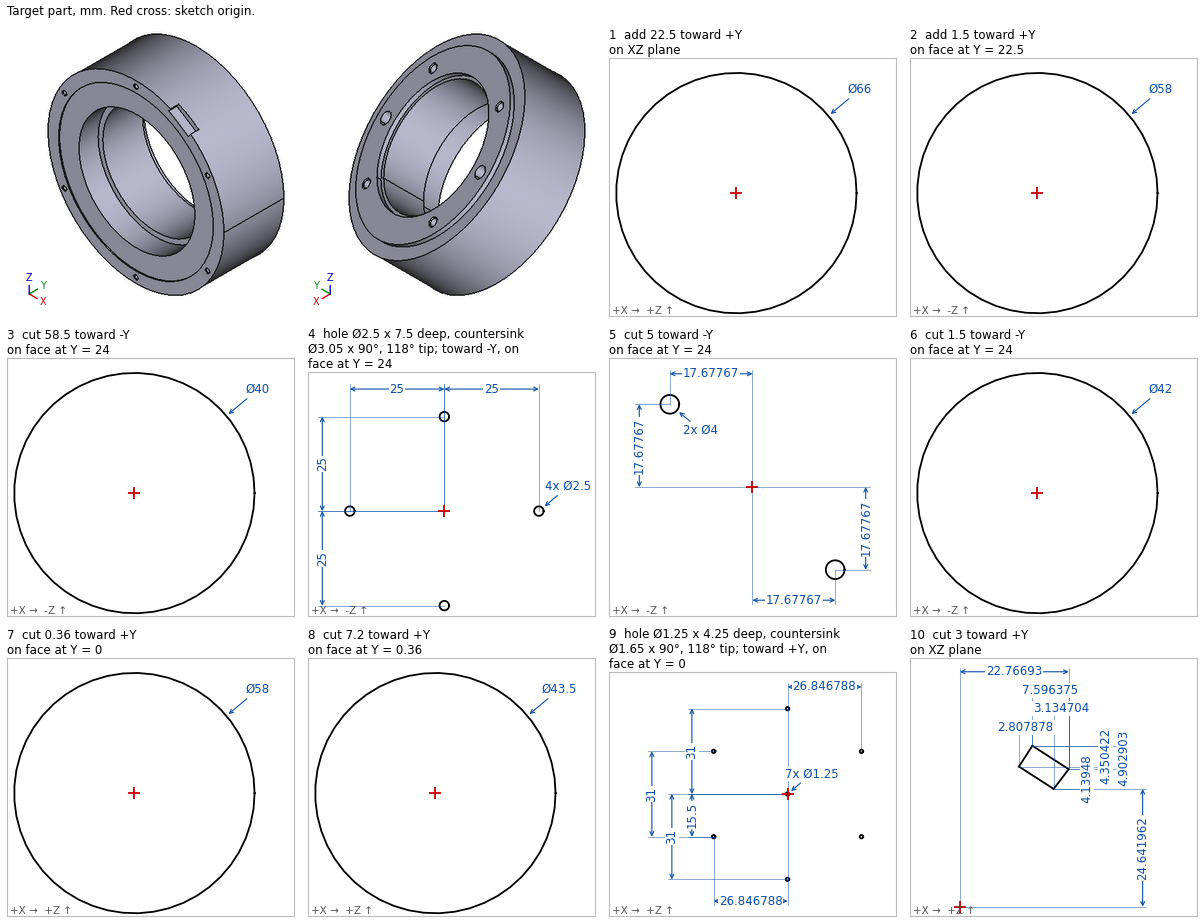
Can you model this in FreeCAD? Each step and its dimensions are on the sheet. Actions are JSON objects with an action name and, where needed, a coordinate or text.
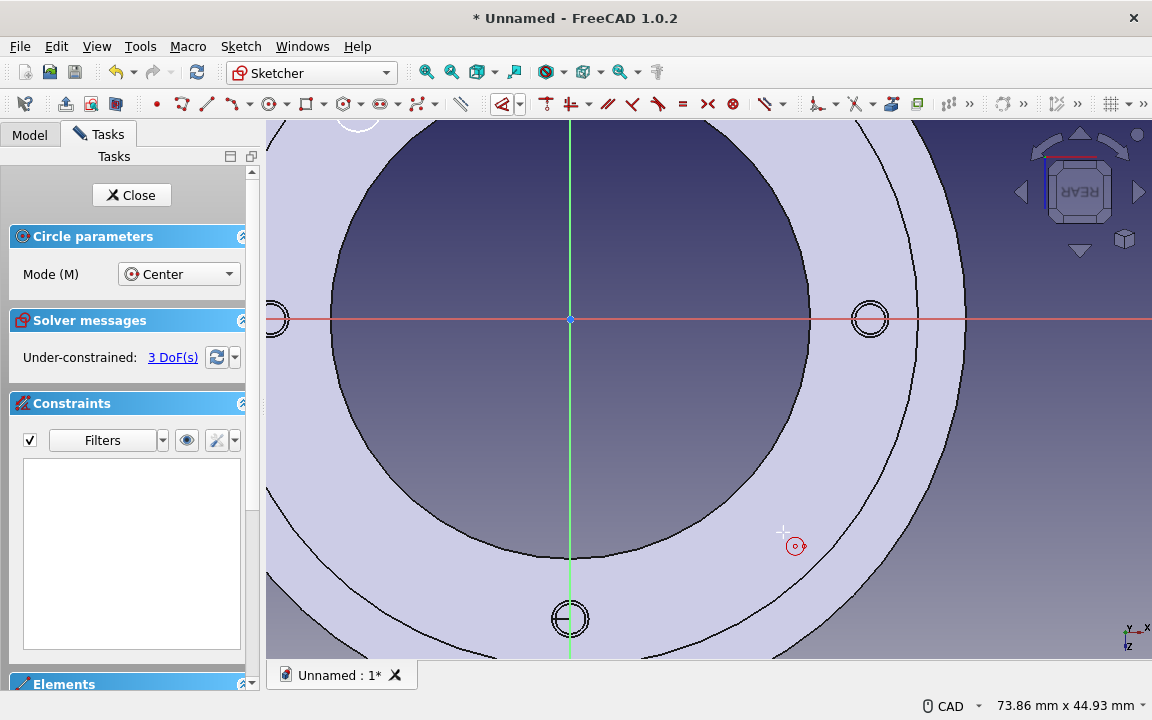
{"action": "left_click", "coordinate": [782, 531]}
{"action": "left_click", "coordinate": [799, 514]}
{"action": "key", "text": "Escape"}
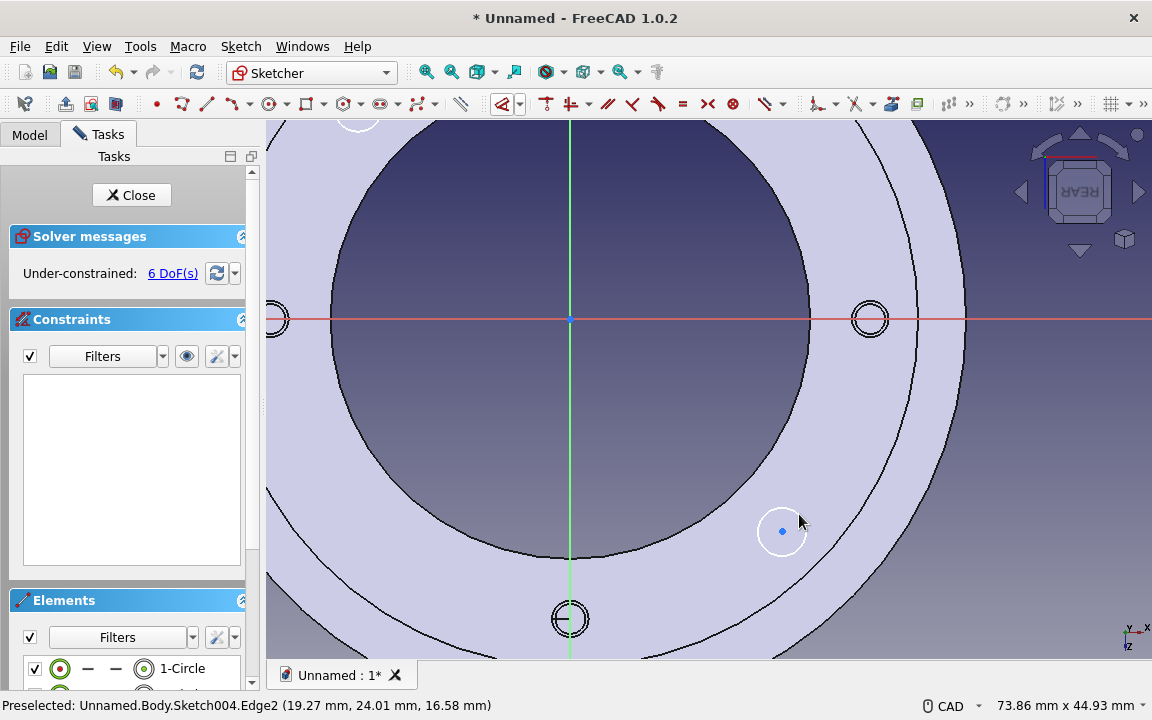
{"action": "scroll", "coordinate": [783, 533], "scroll_direction": "down", "scroll_amount": 2}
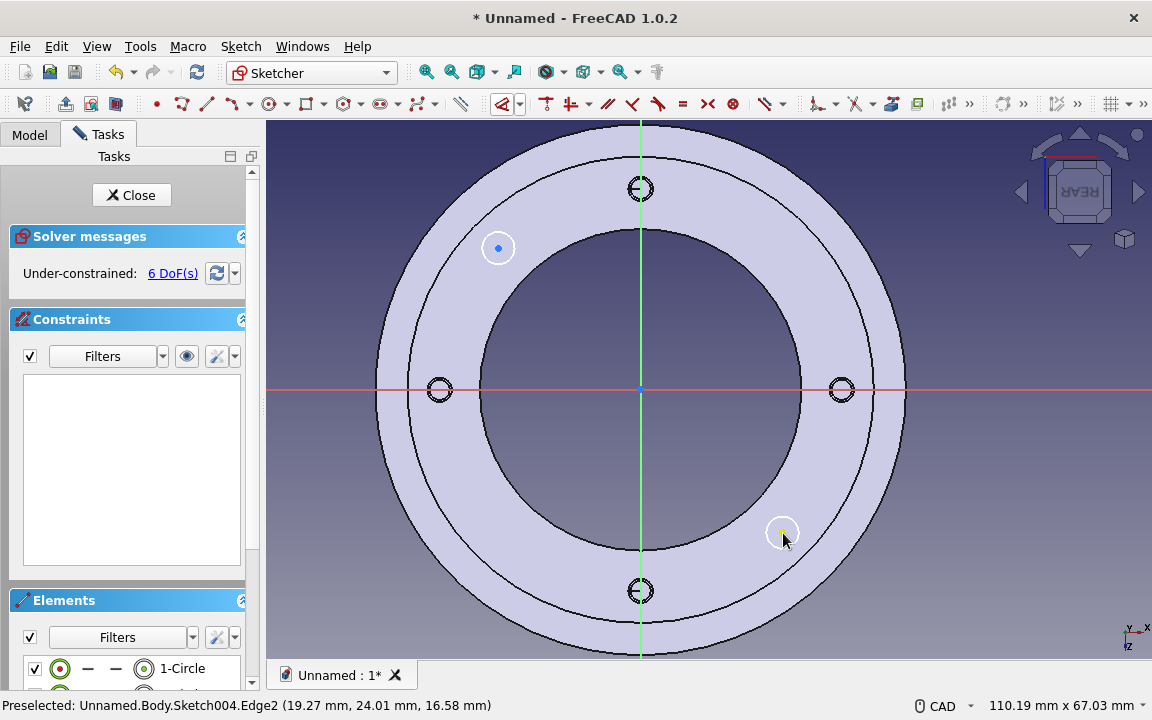
{"action": "left_click", "coordinate": [510, 237]}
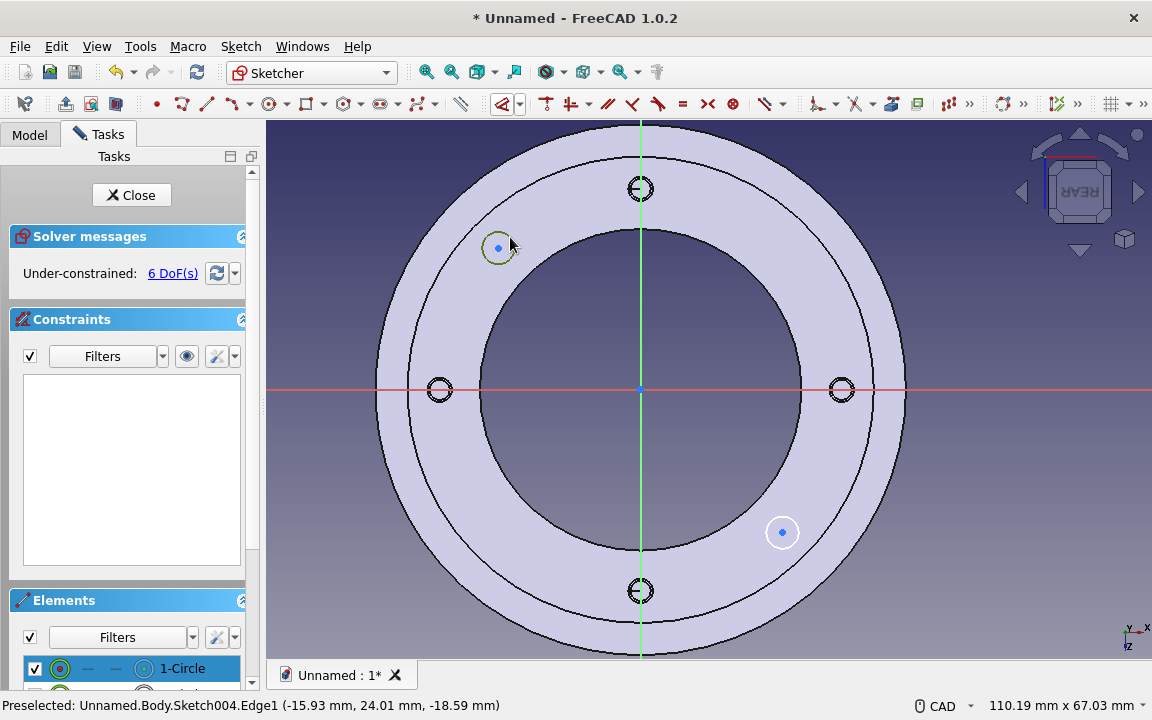
{"action": "left_click", "coordinate": [794, 521]}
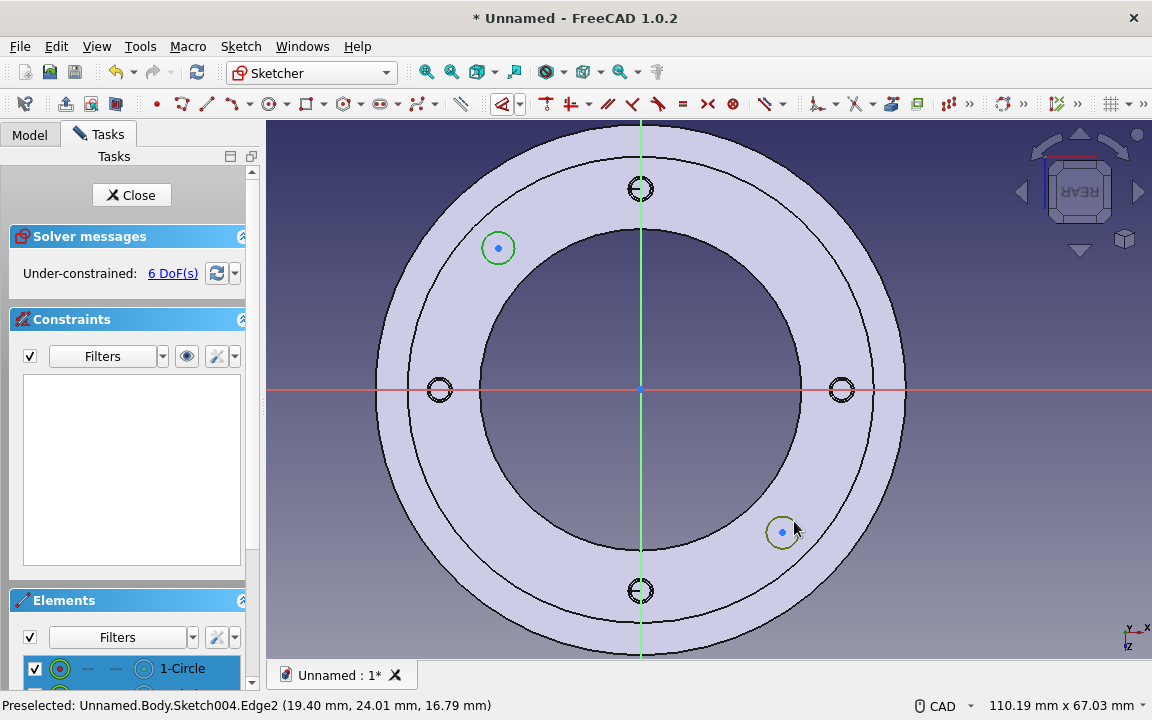
{"action": "left_click", "coordinate": [683, 104]}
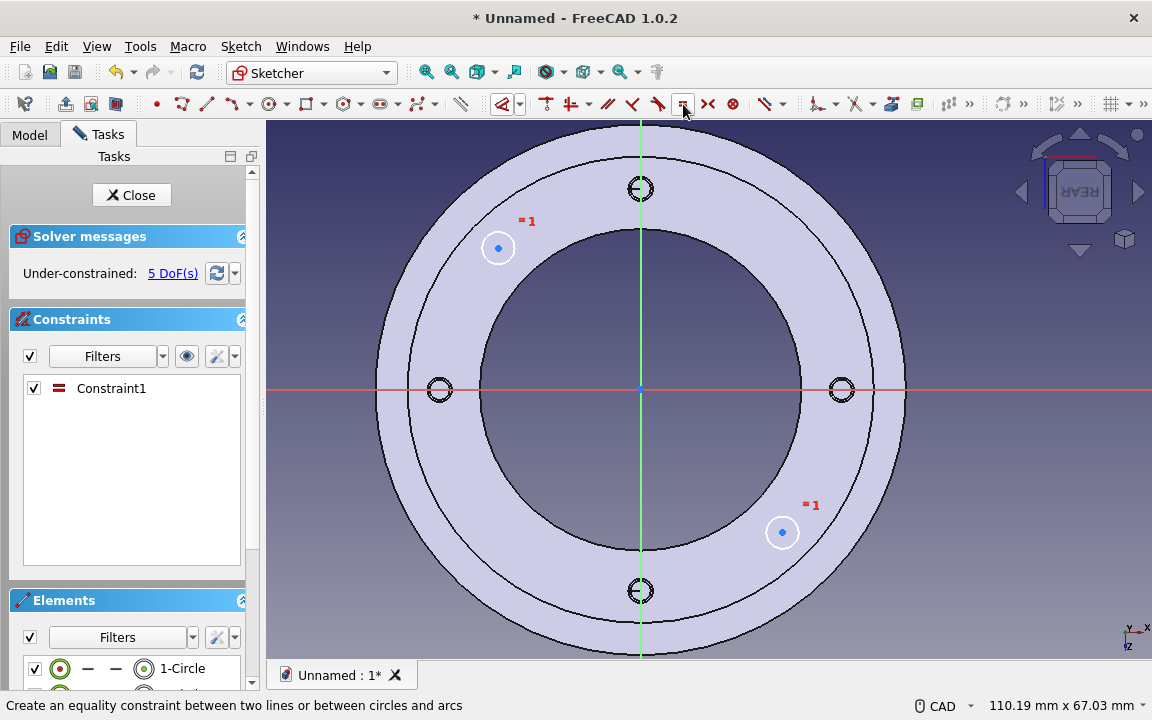
{"action": "scroll", "coordinate": [510, 237], "scroll_direction": "up", "scroll_amount": 2}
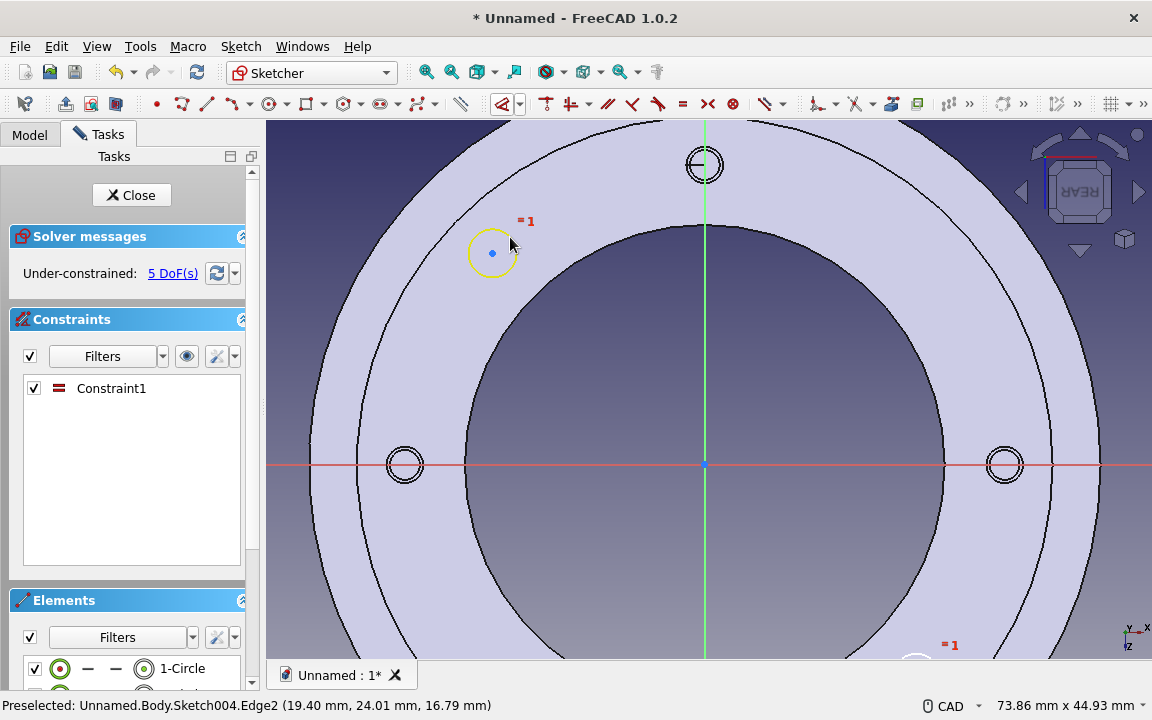
{"action": "left_click", "coordinate": [510, 236]}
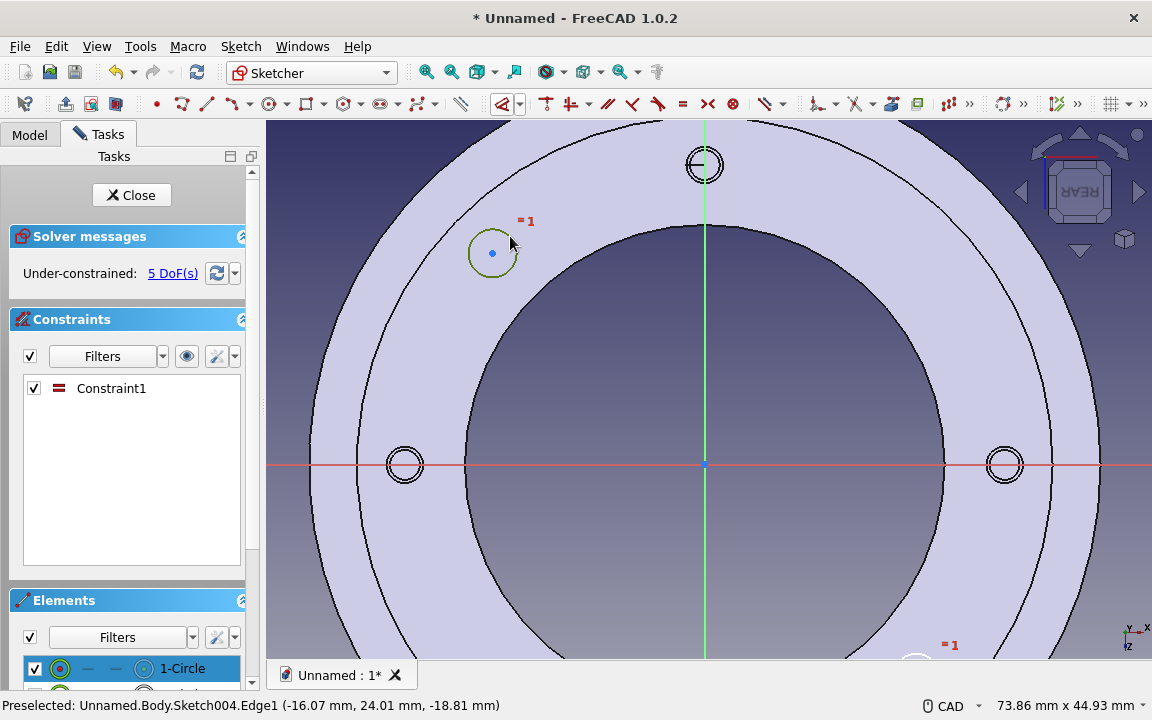
{"action": "key", "text": "k o"}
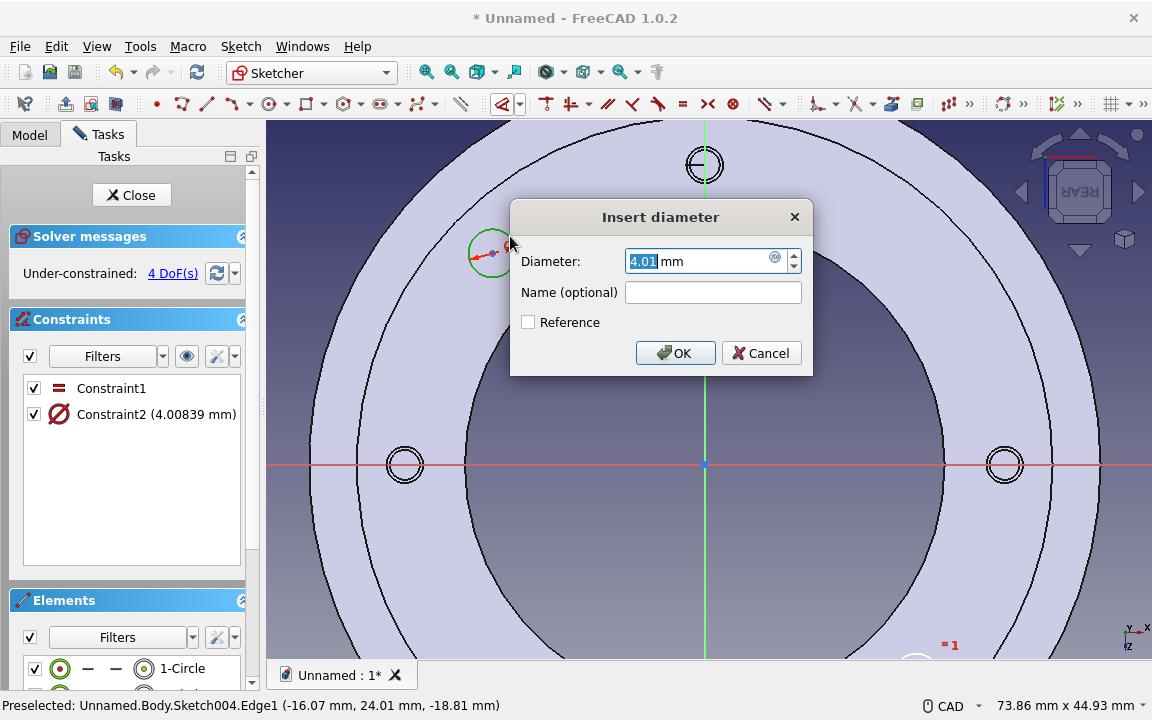
{"action": "type", "text": "4"}
{"action": "key", "text": "Return"}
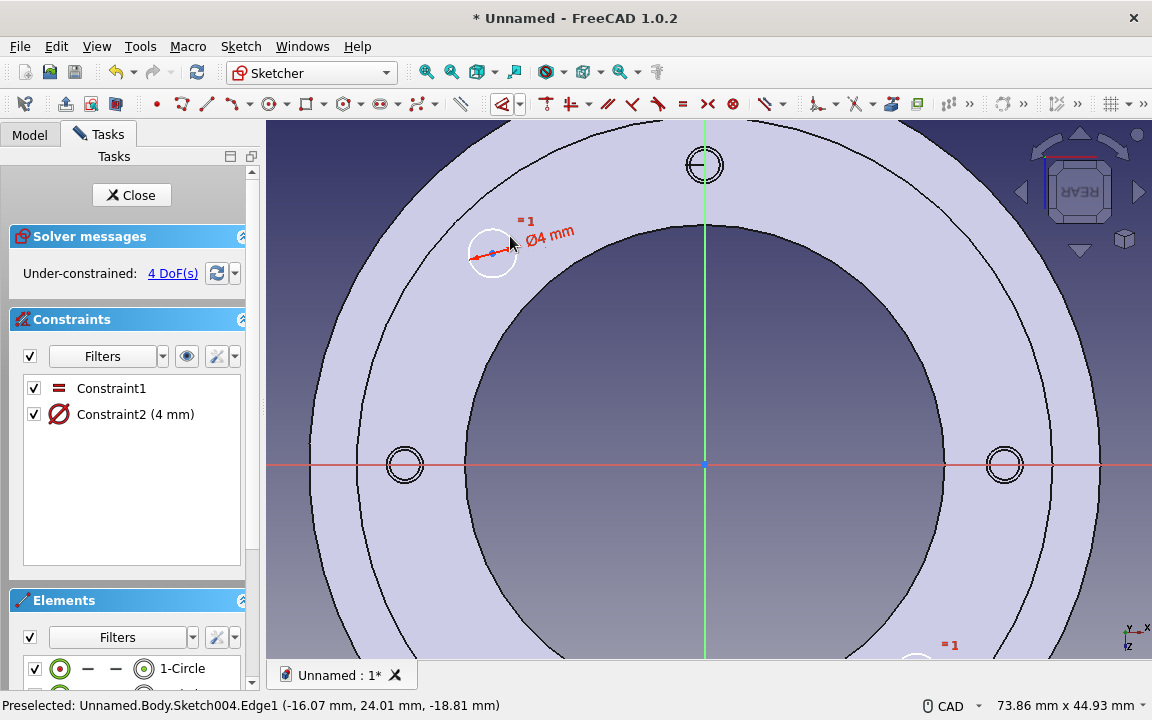
{"action": "left_click", "coordinate": [493, 253]}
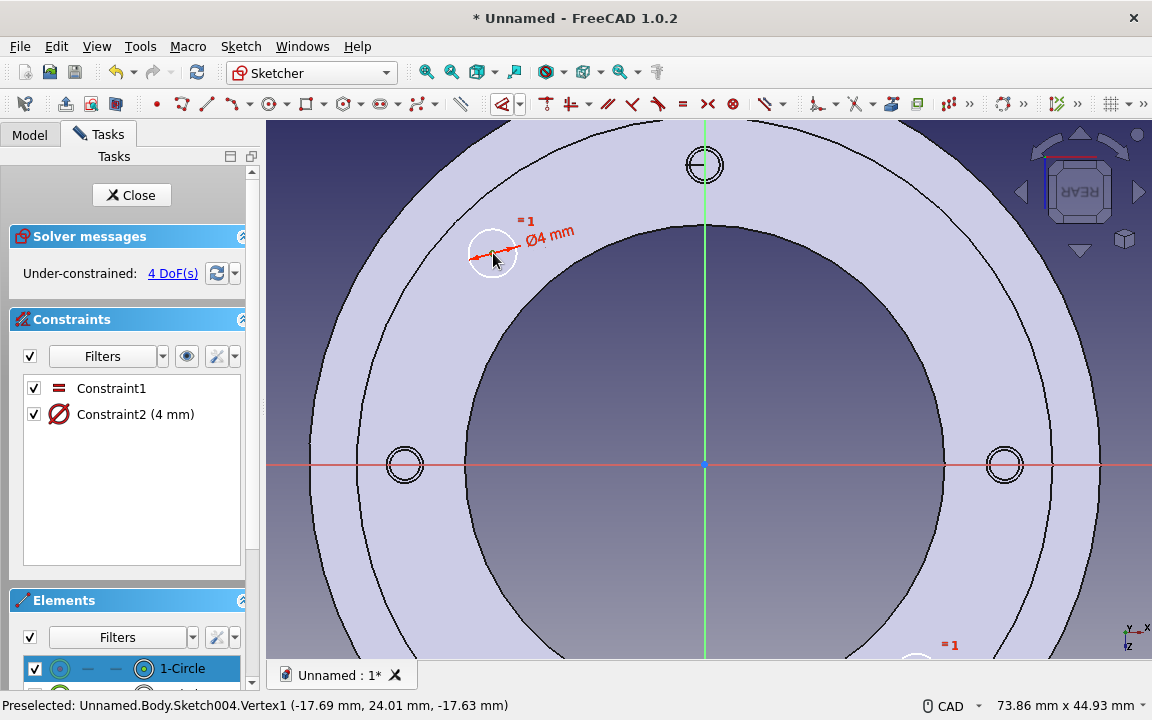
{"action": "left_click", "coordinate": [520, 104]}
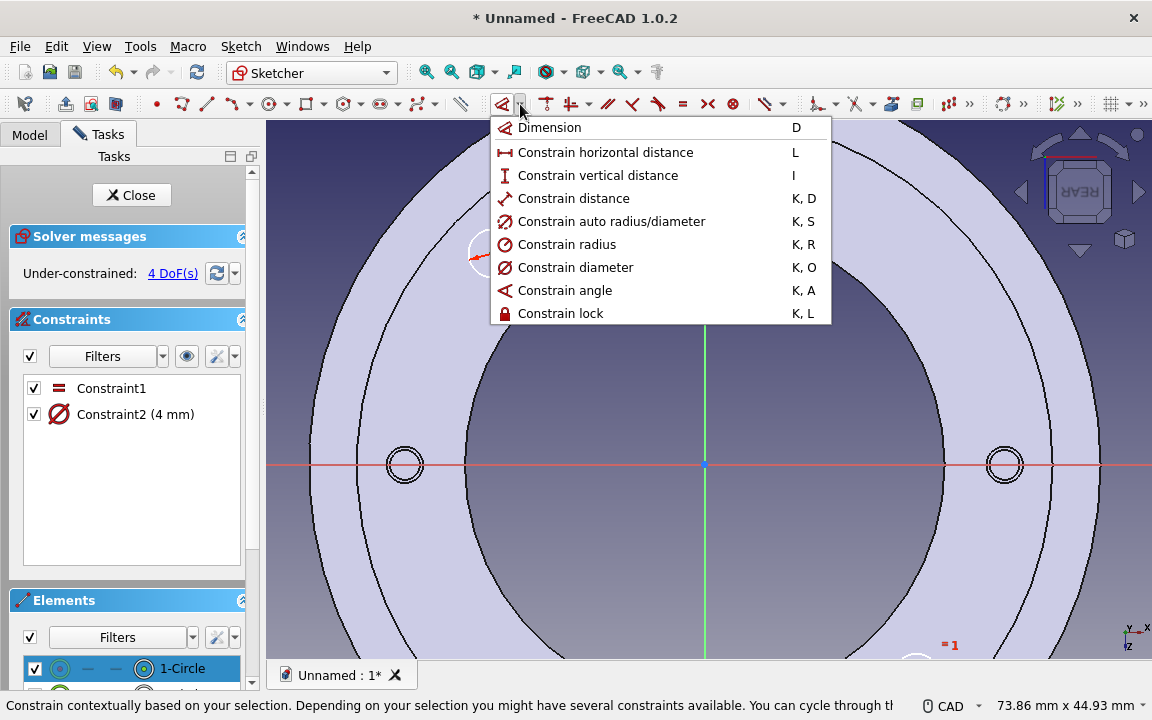
{"action": "left_click", "coordinate": [661, 152]}